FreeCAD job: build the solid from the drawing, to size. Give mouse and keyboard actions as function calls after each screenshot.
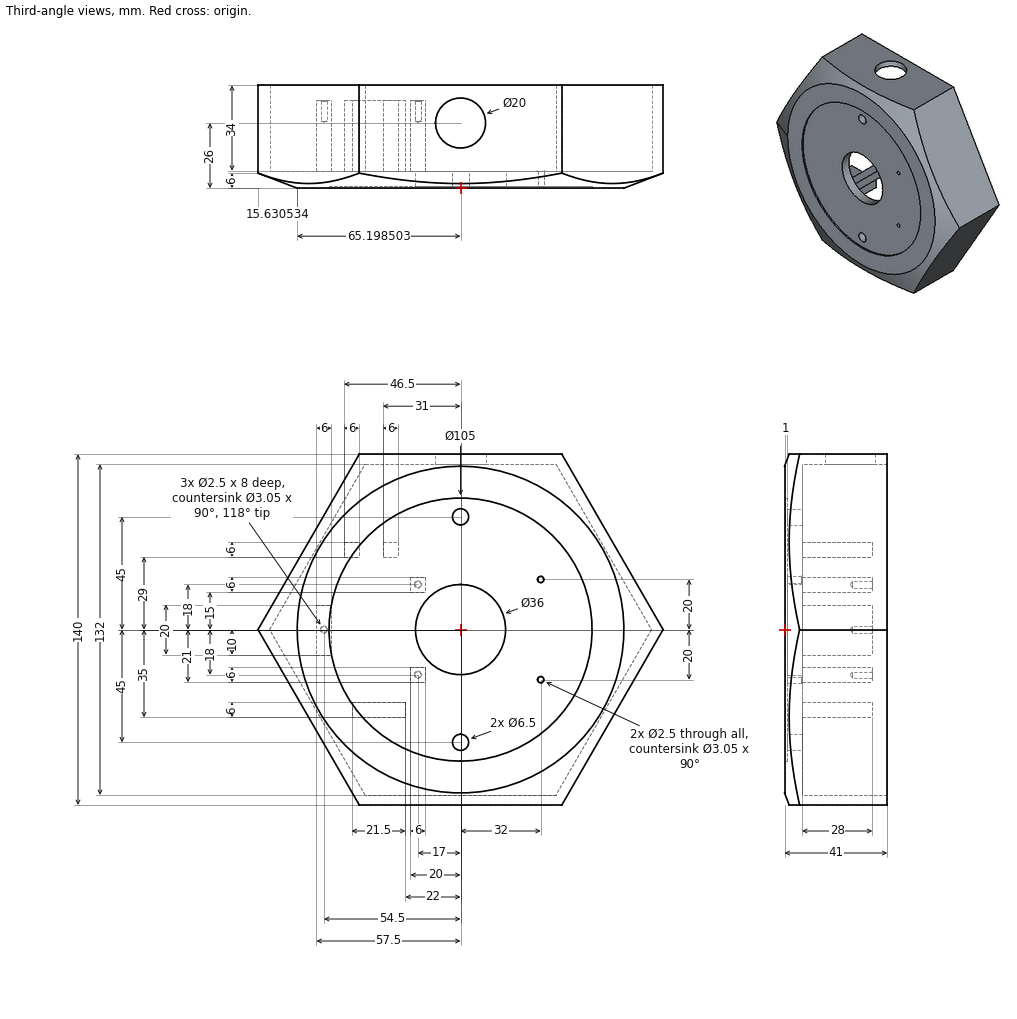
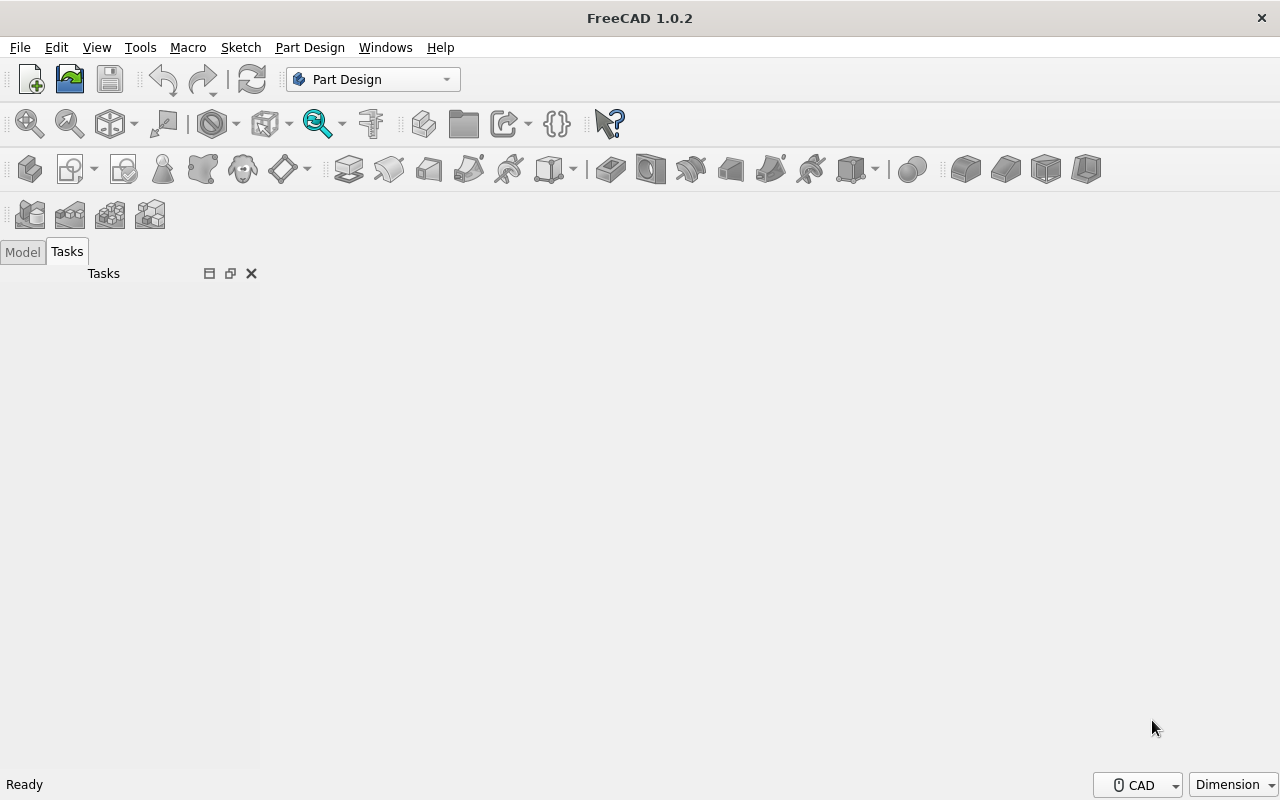
key(ctrl+n)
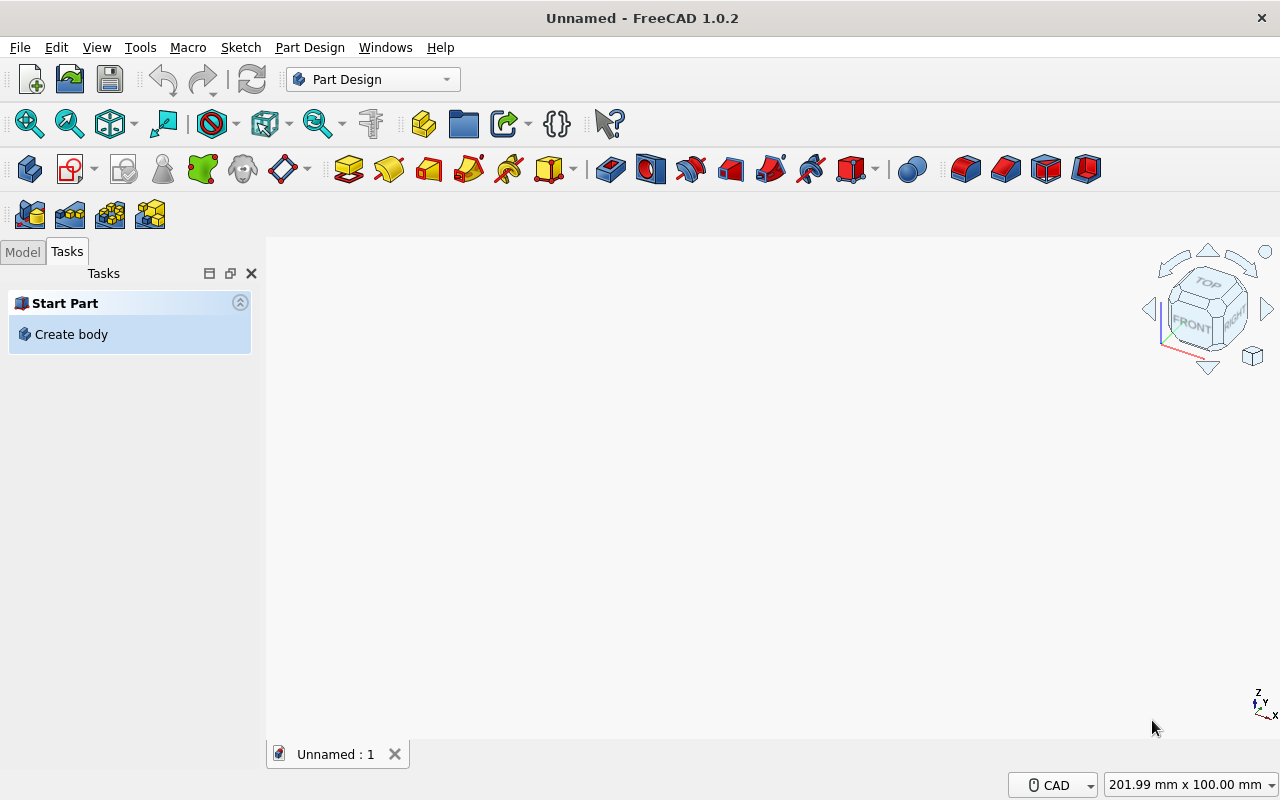
click(70, 170)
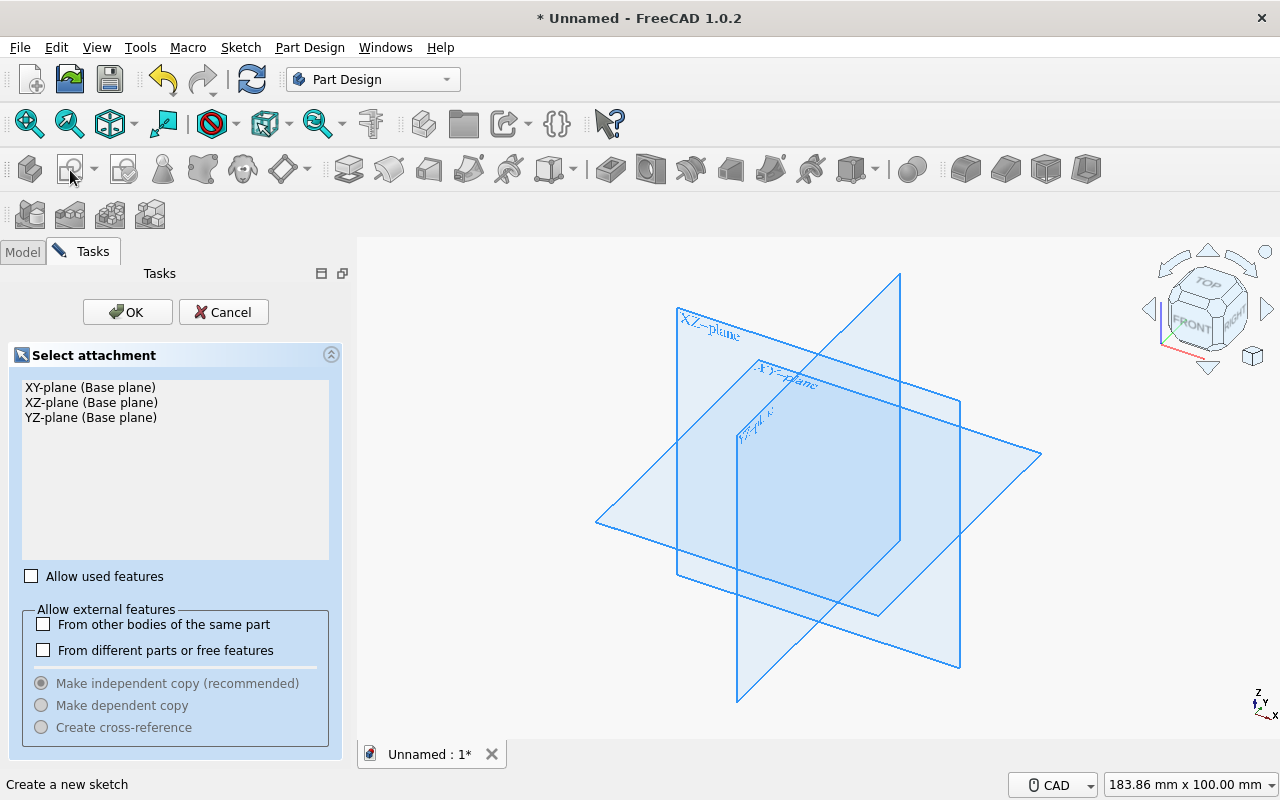
click(82, 402)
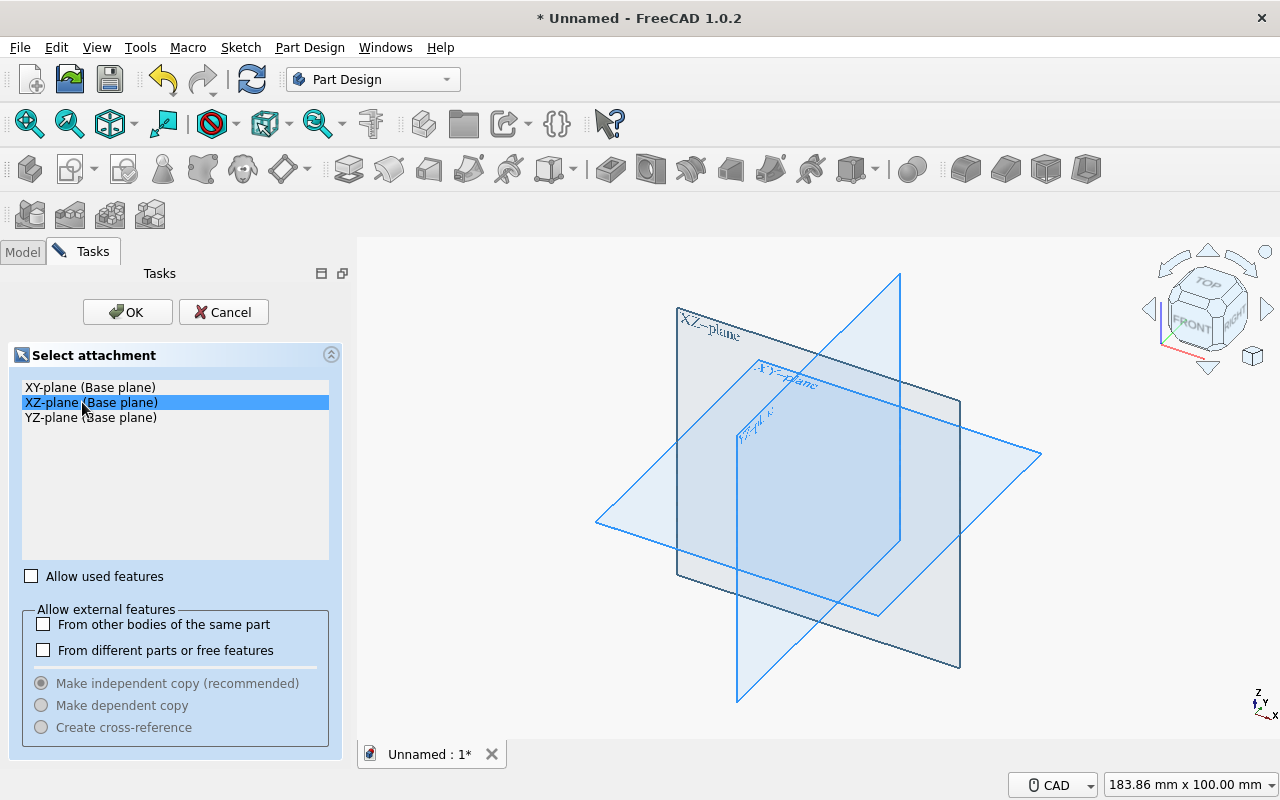
click(128, 312)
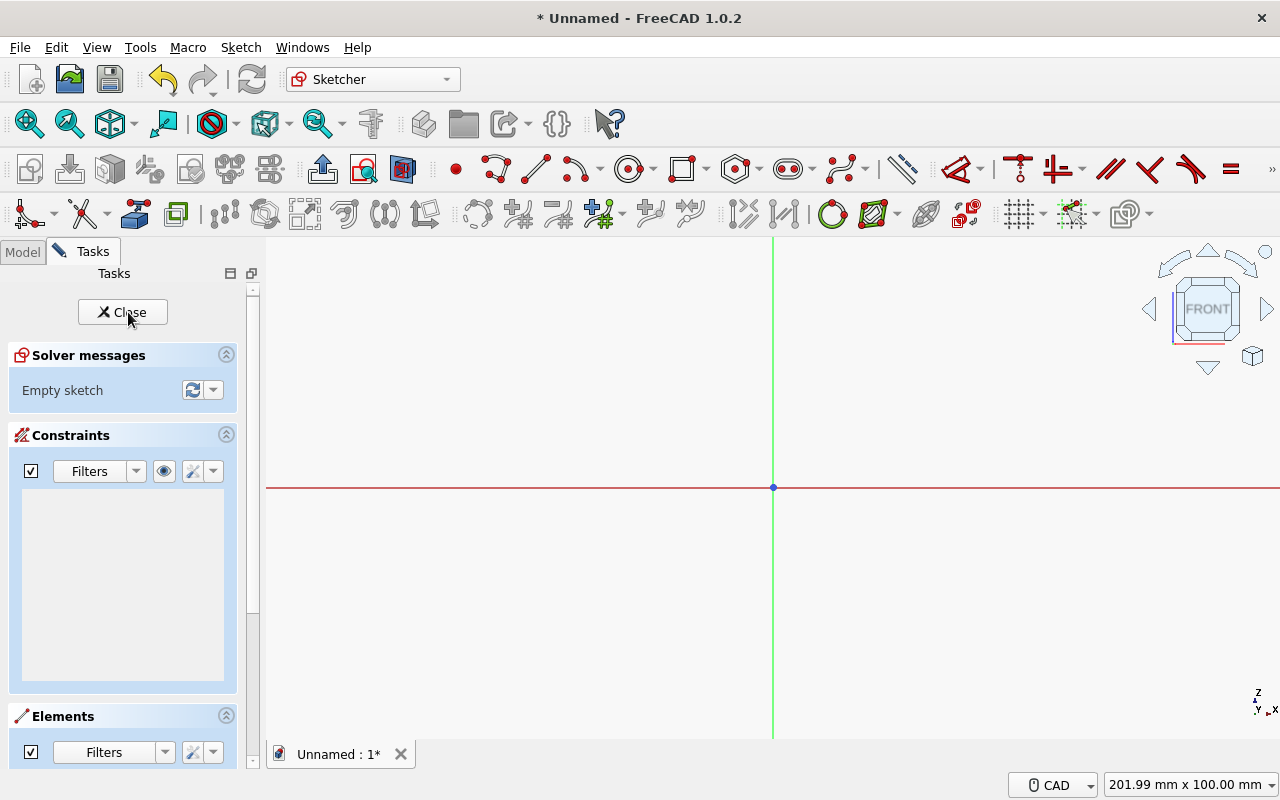
scroll(649, 488, down, 4)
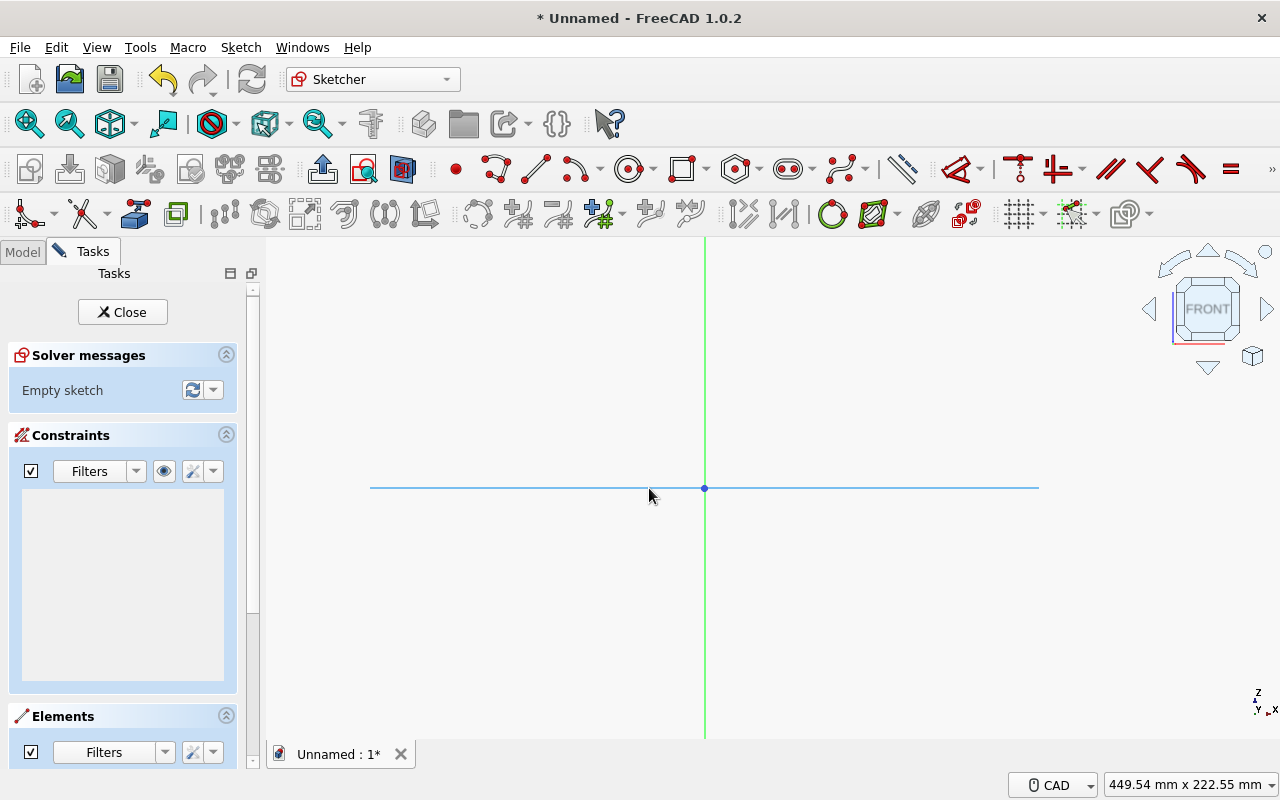
key(g)
key(p)
key(6)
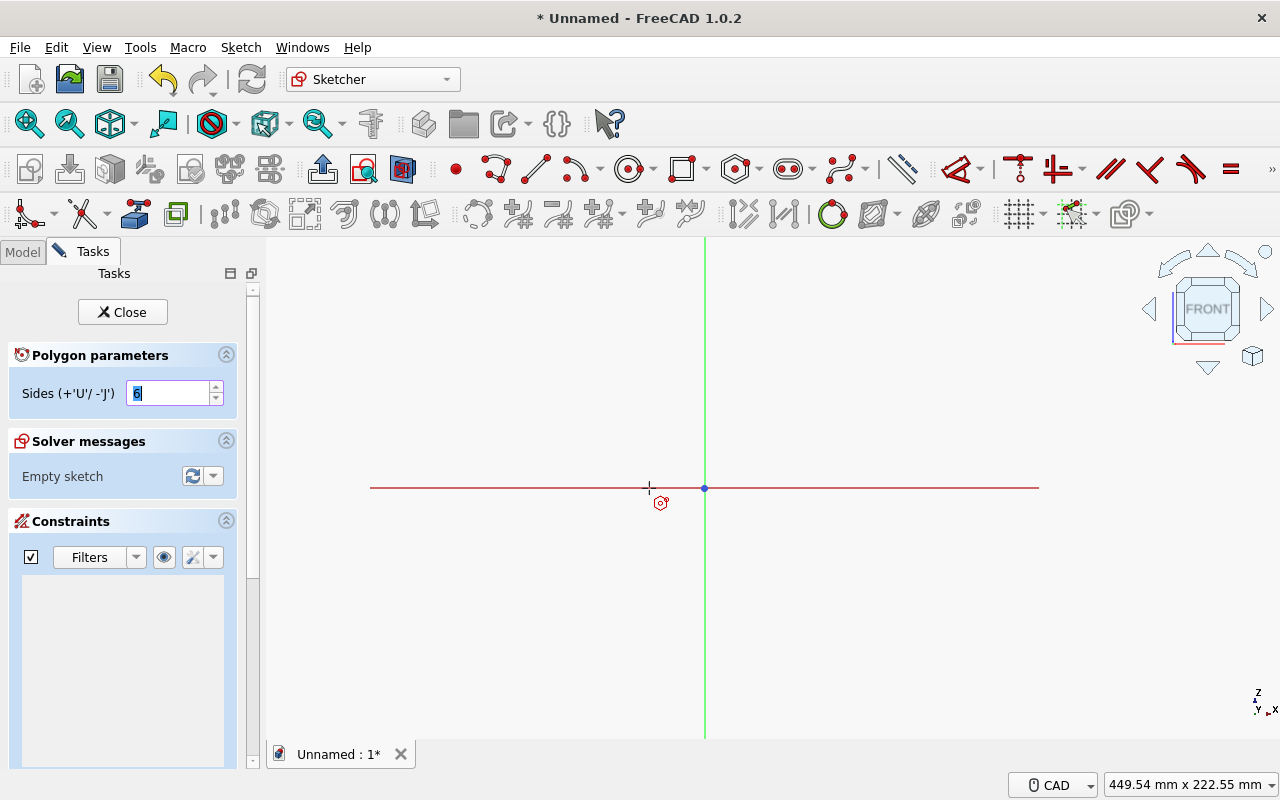
click(705, 488)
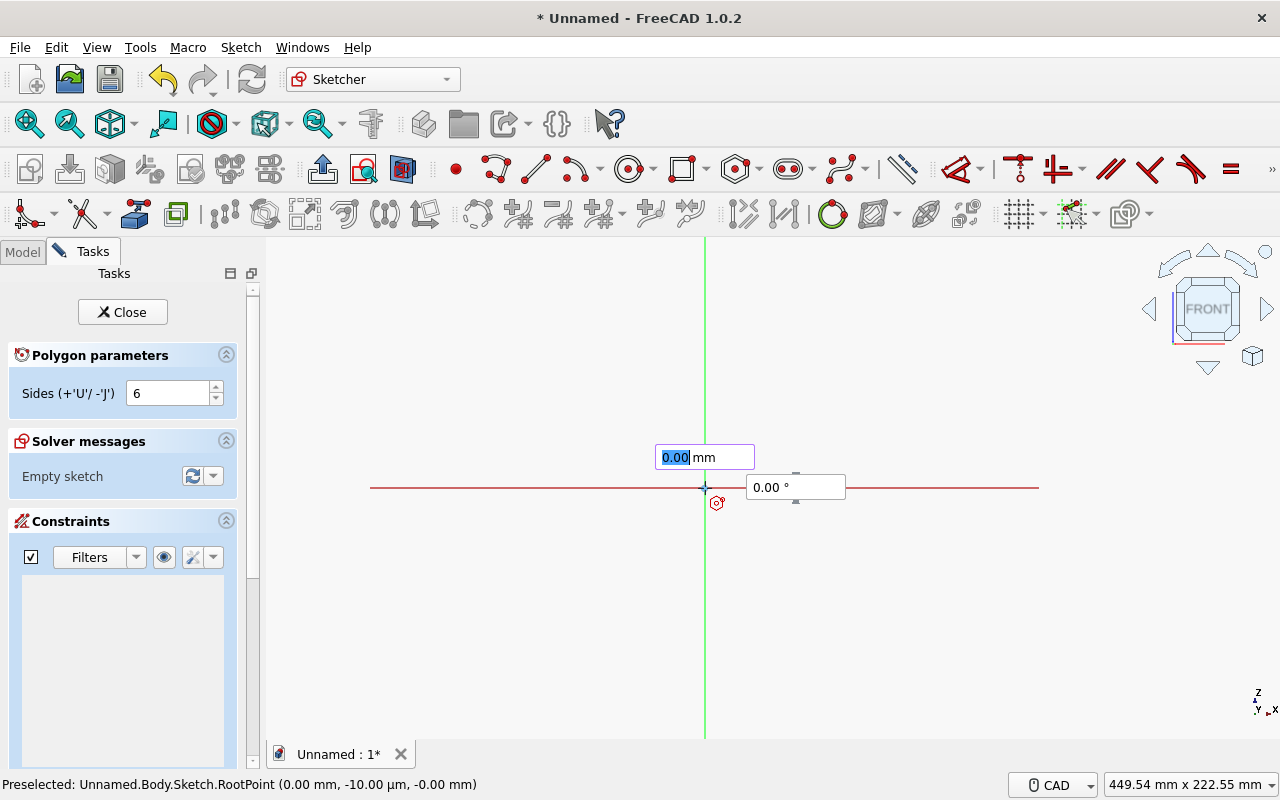
click(523, 488)
right_click(523, 488)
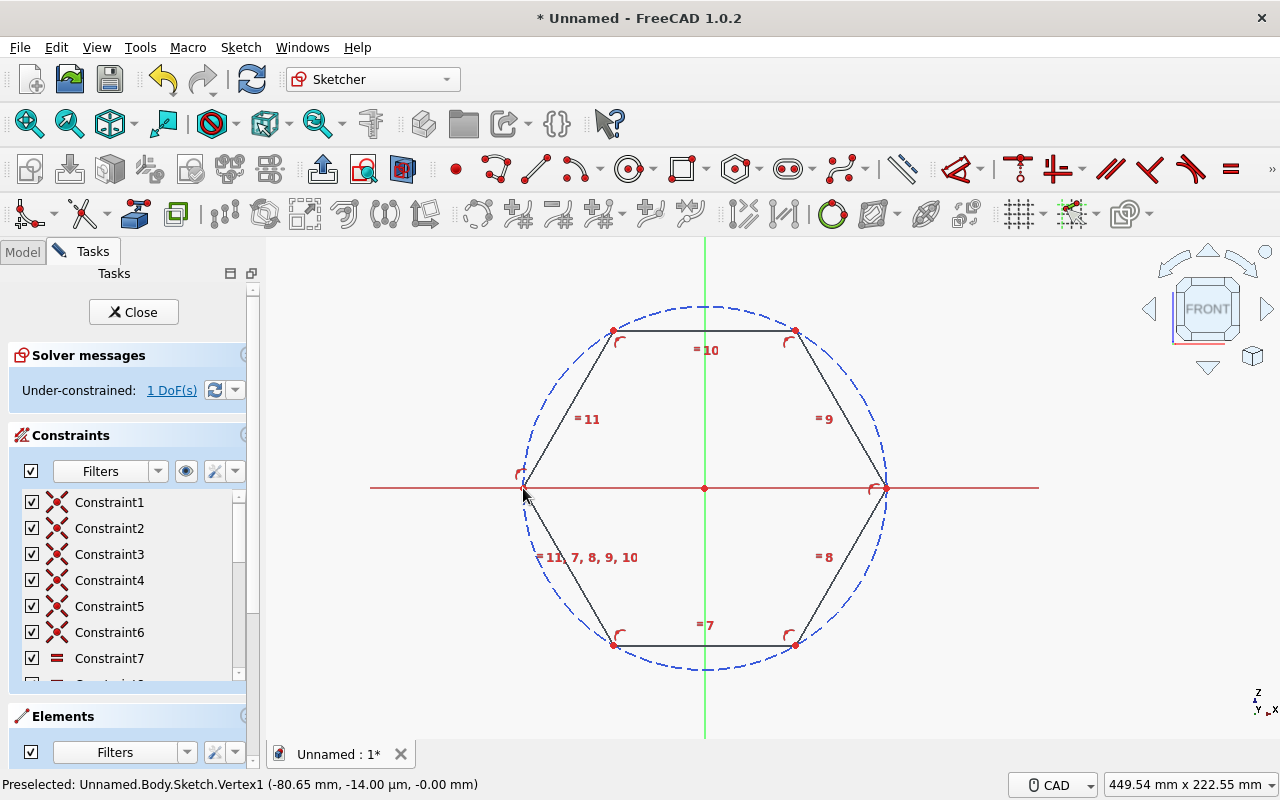
click(614, 646)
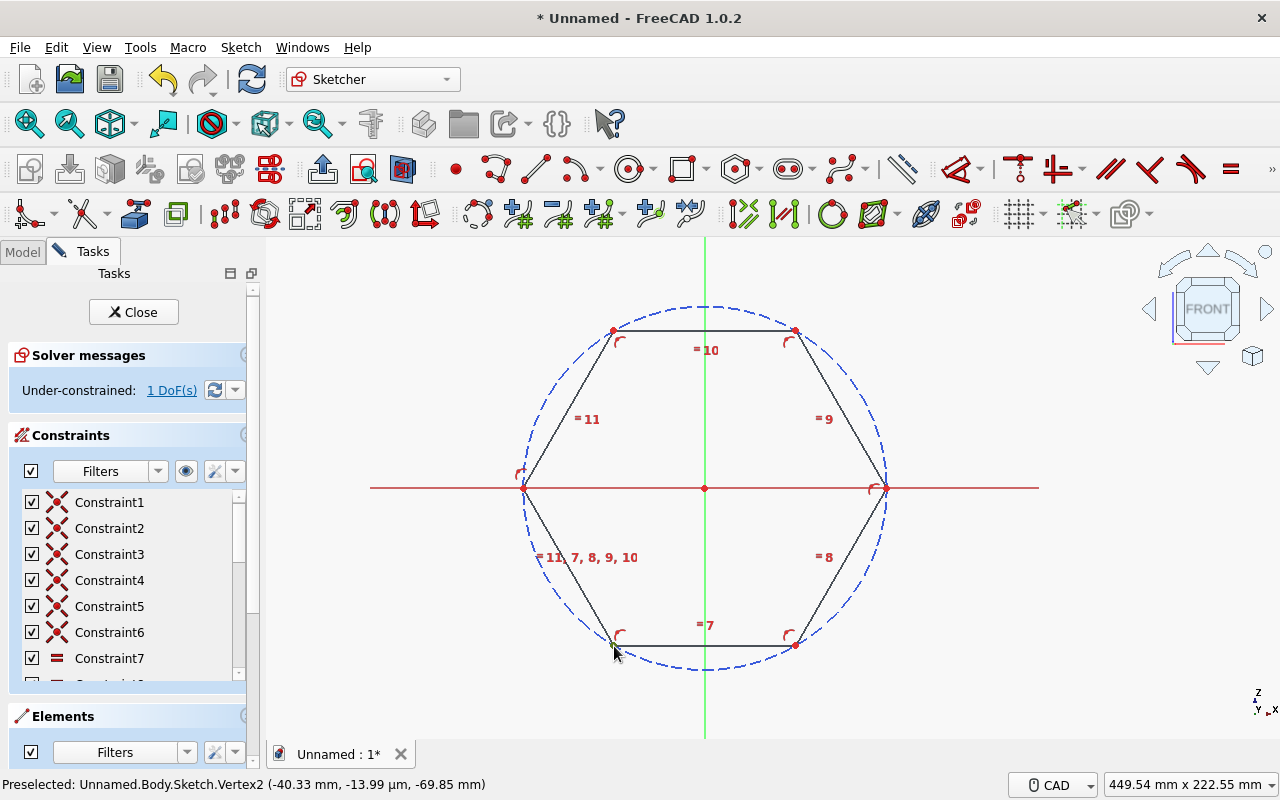
click(796, 331)